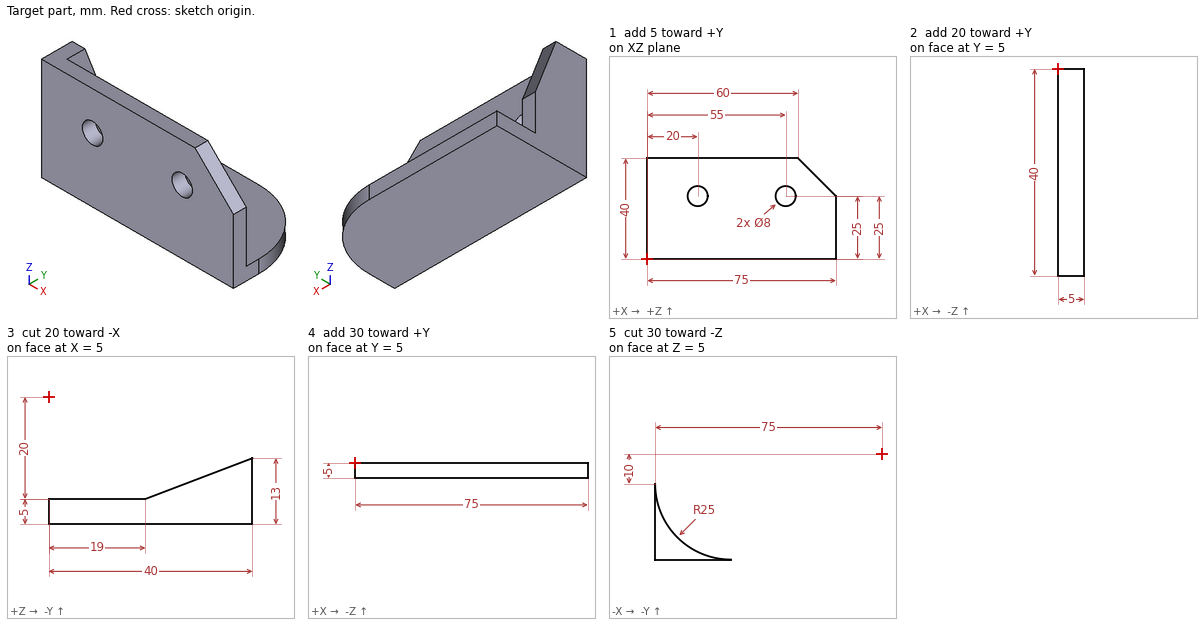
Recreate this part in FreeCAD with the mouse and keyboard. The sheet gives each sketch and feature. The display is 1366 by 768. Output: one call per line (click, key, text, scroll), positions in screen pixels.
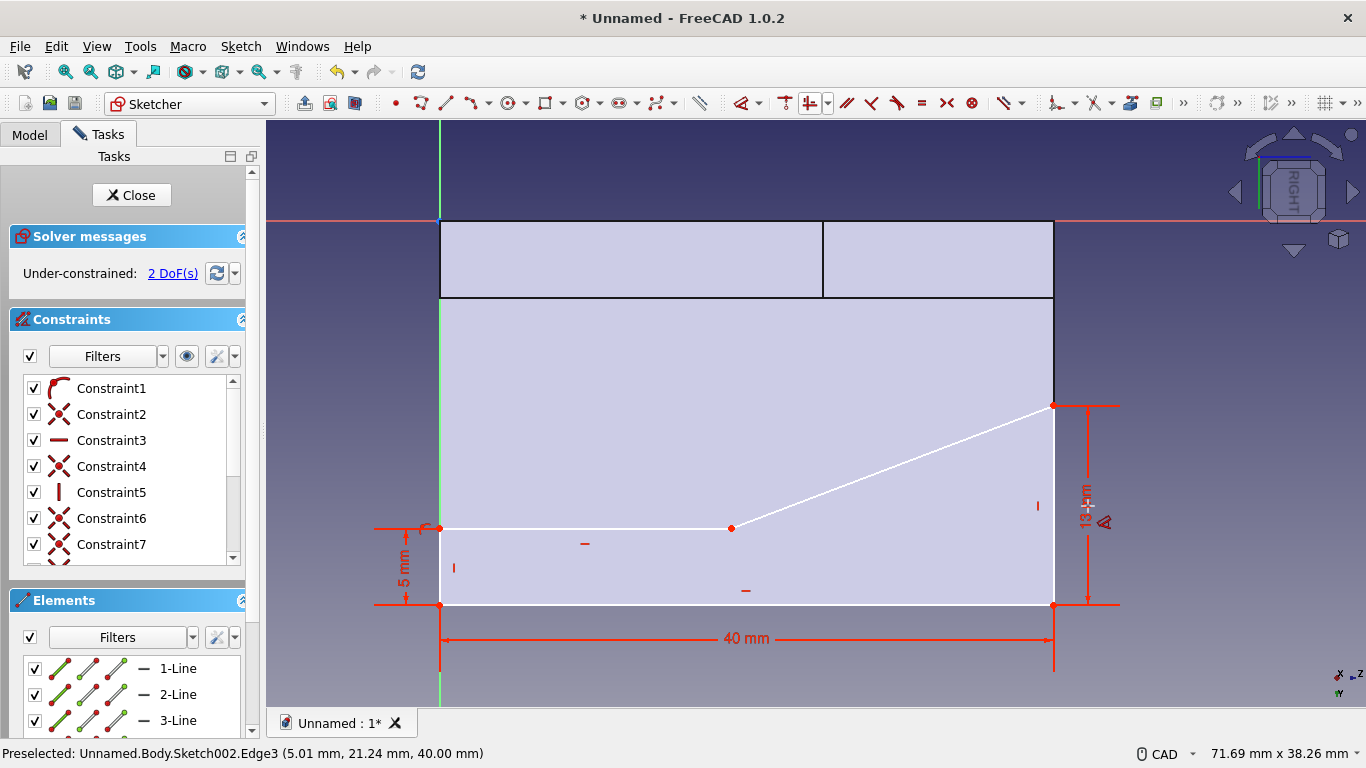
click(644, 529)
click(585, 563)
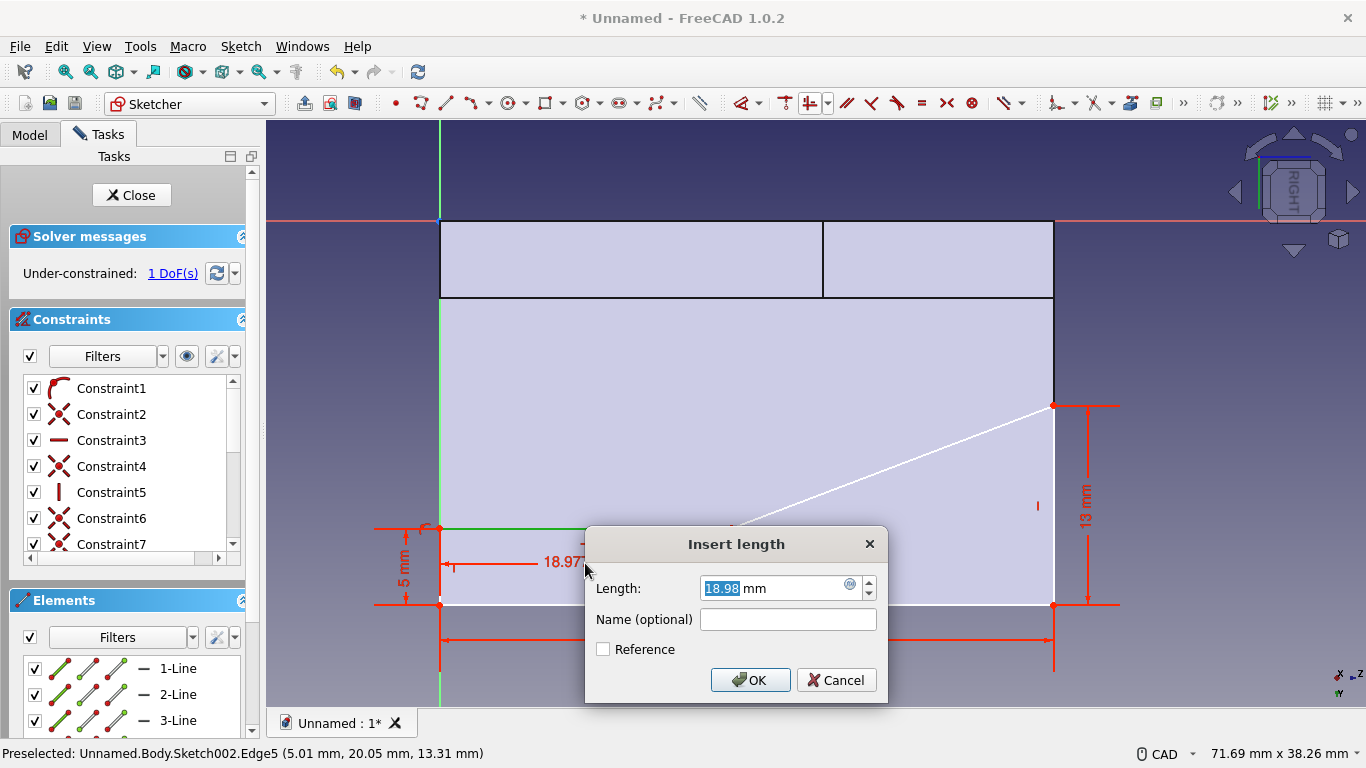
text(19)
key(Return)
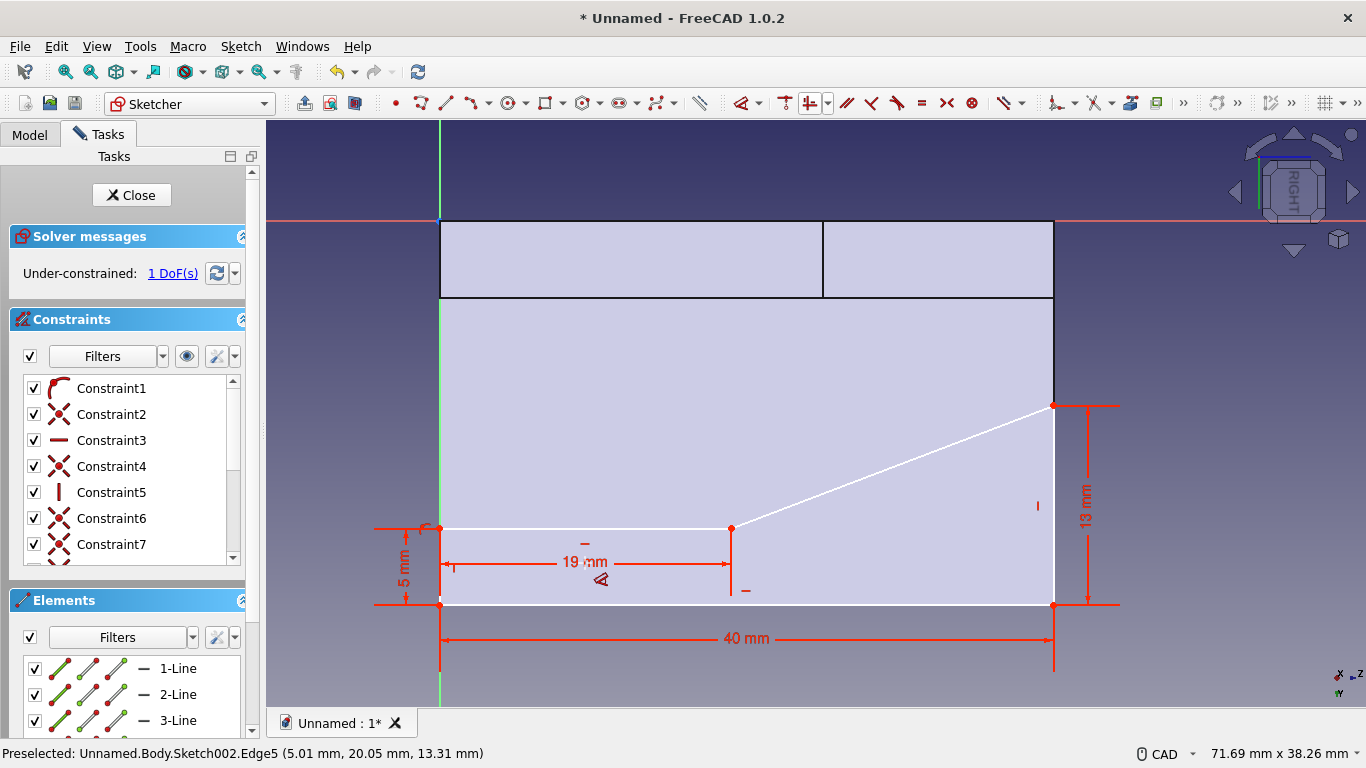
click(440, 529)
click(406, 375)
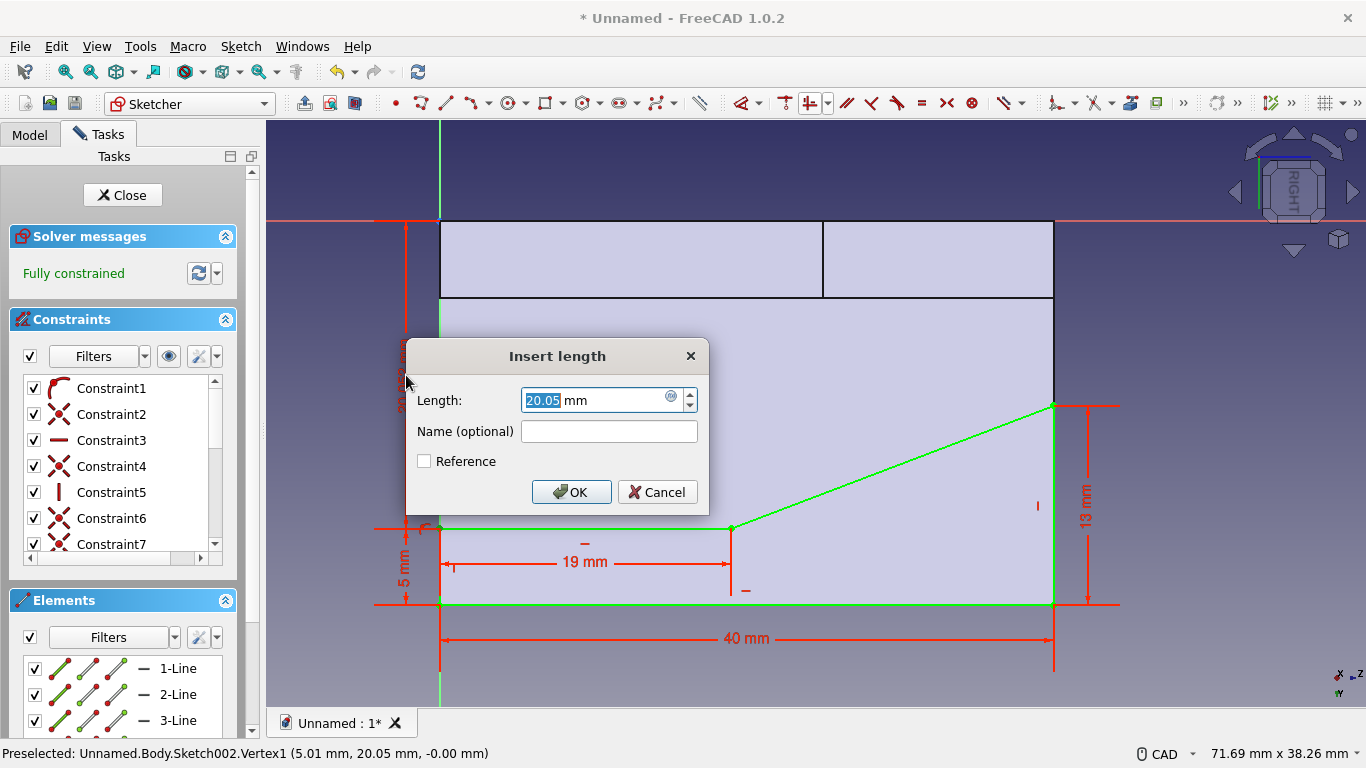
text(20)
key(Return)
key(Escape)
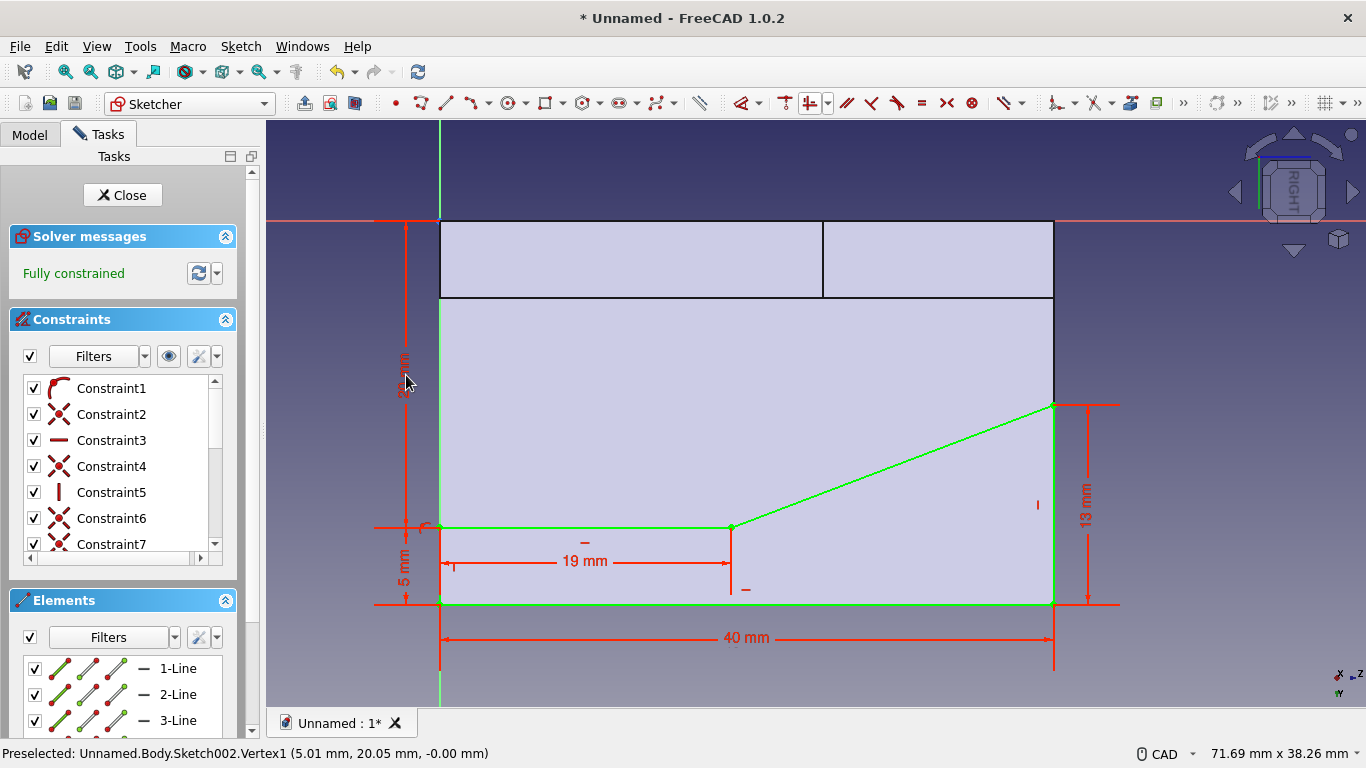
click(123, 195)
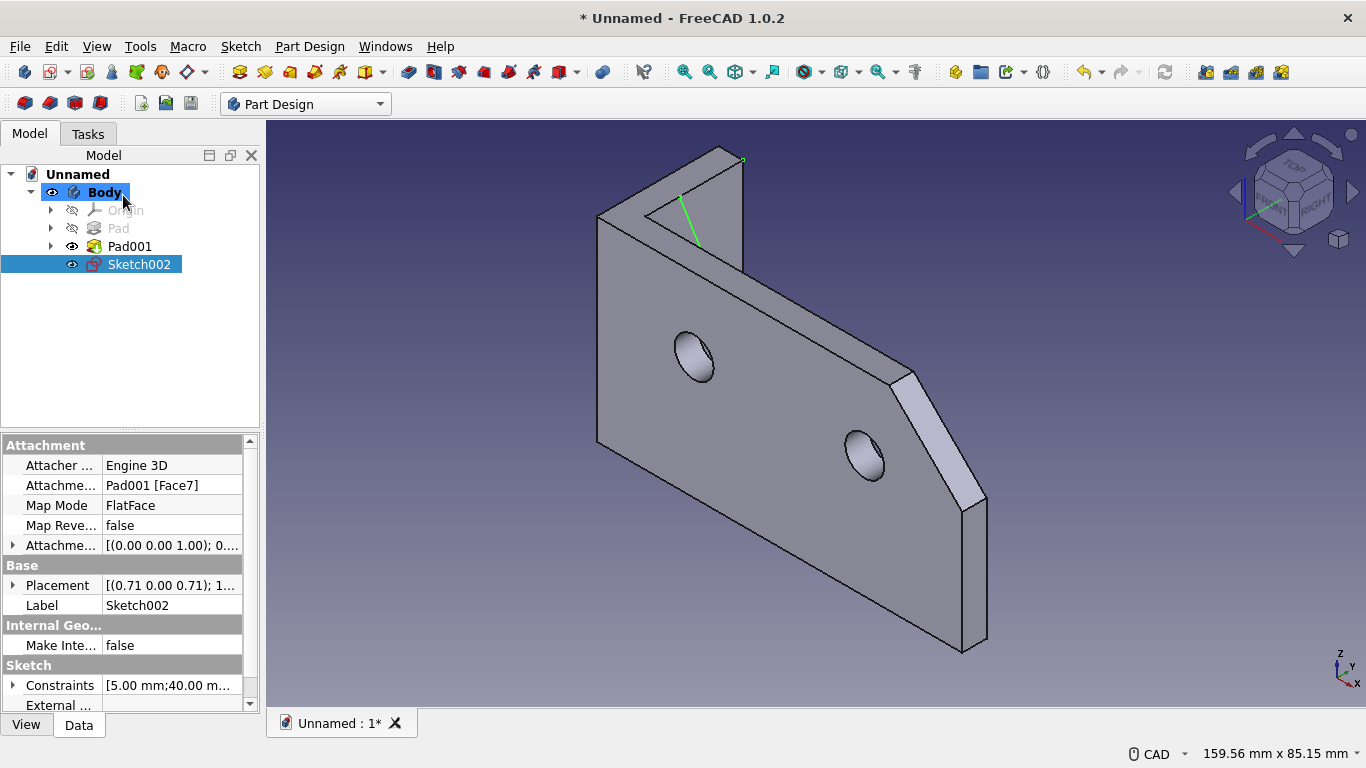
click(409, 72)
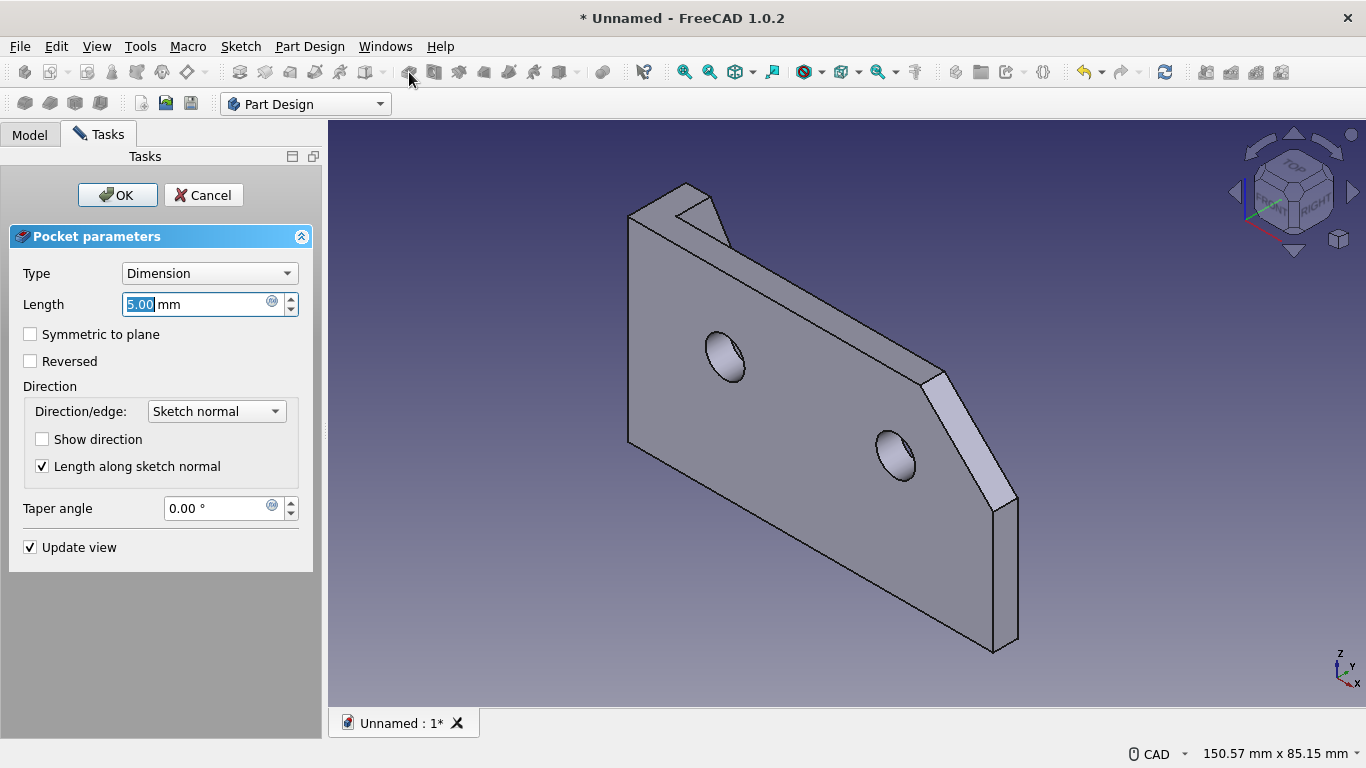
text(20)
key(Tab)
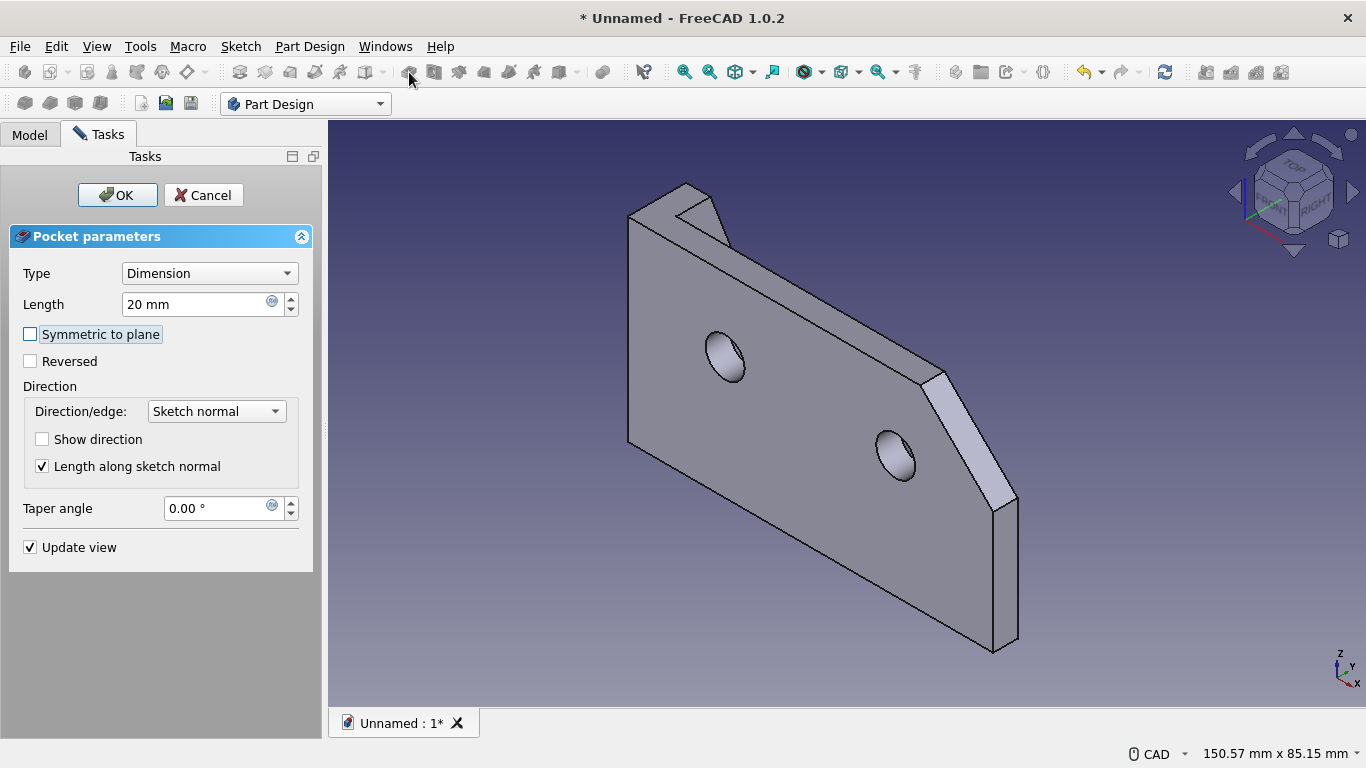
click(118, 195)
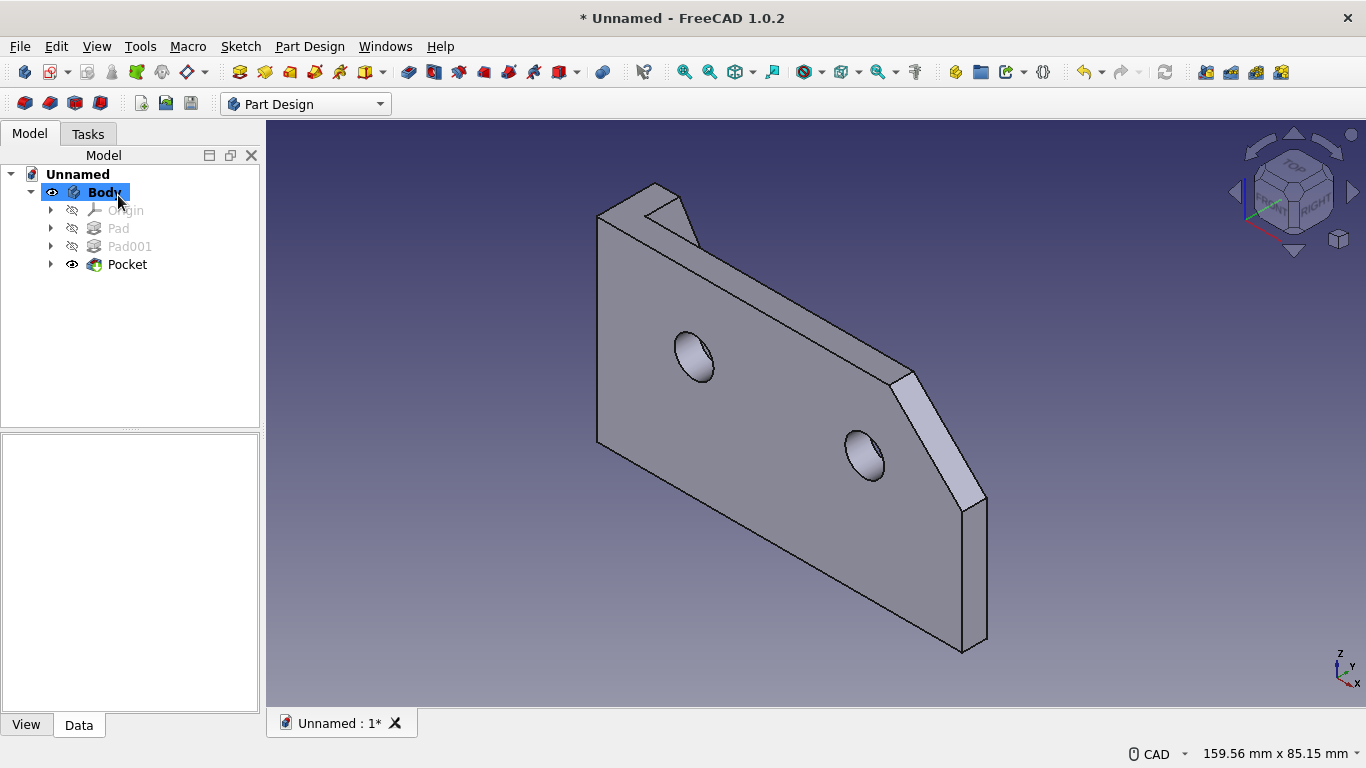
key(4)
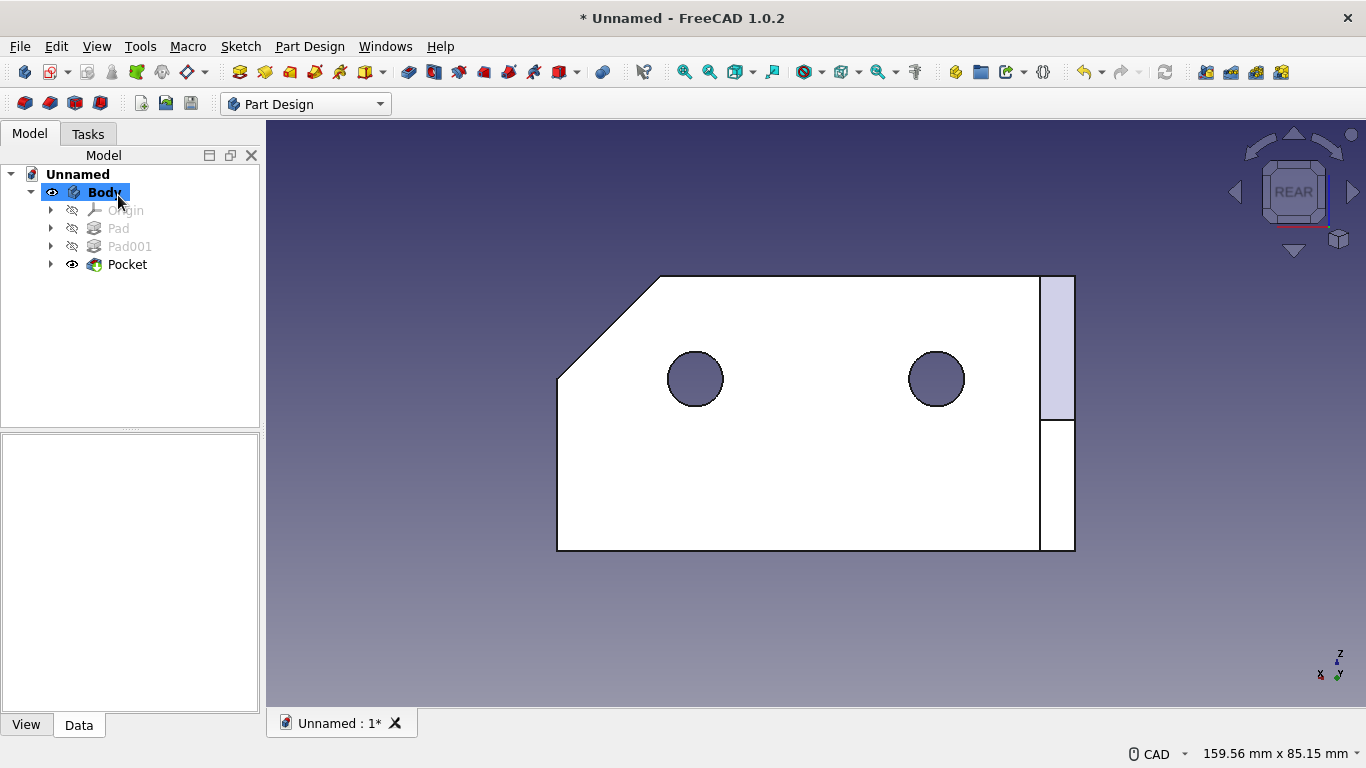
click(799, 452)